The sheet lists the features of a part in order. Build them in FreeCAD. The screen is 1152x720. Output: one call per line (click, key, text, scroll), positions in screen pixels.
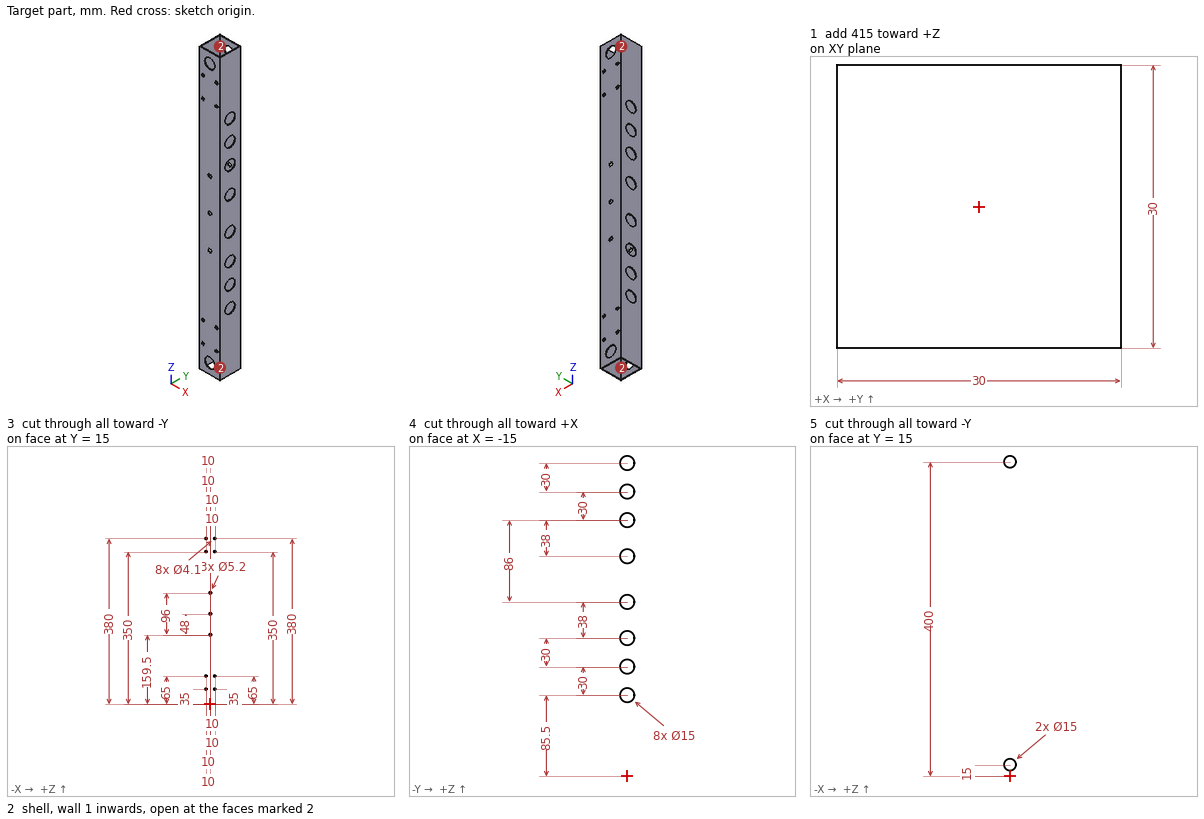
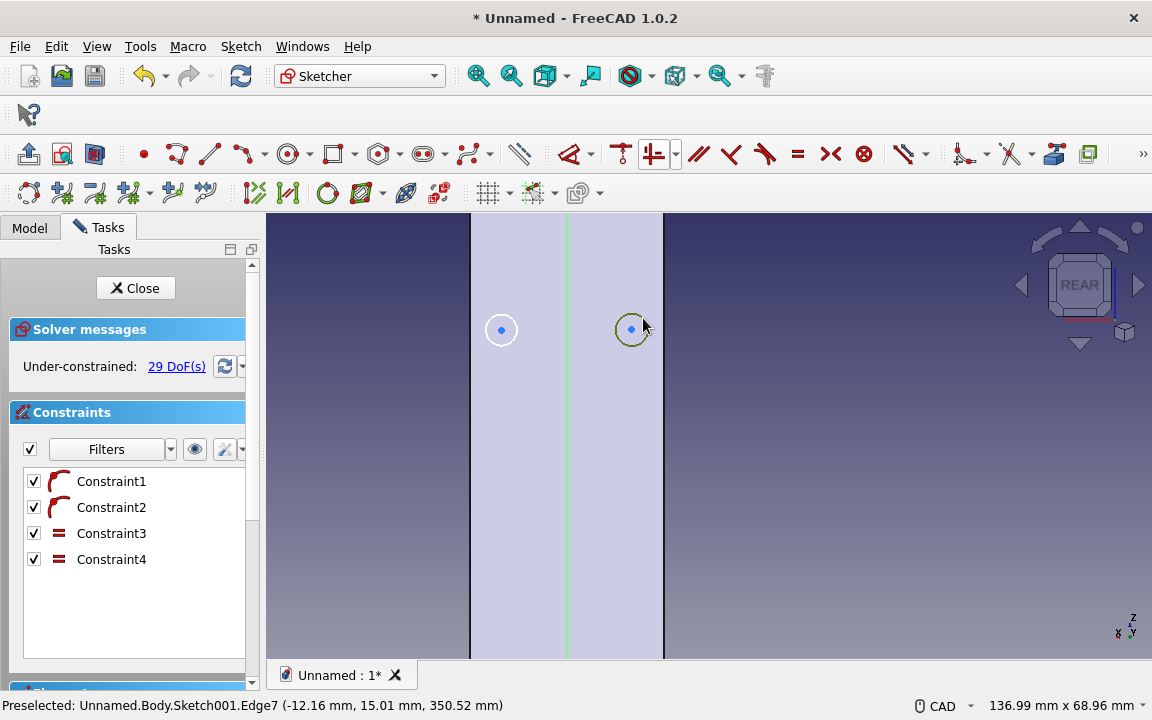
scroll(650, 322, down, 11)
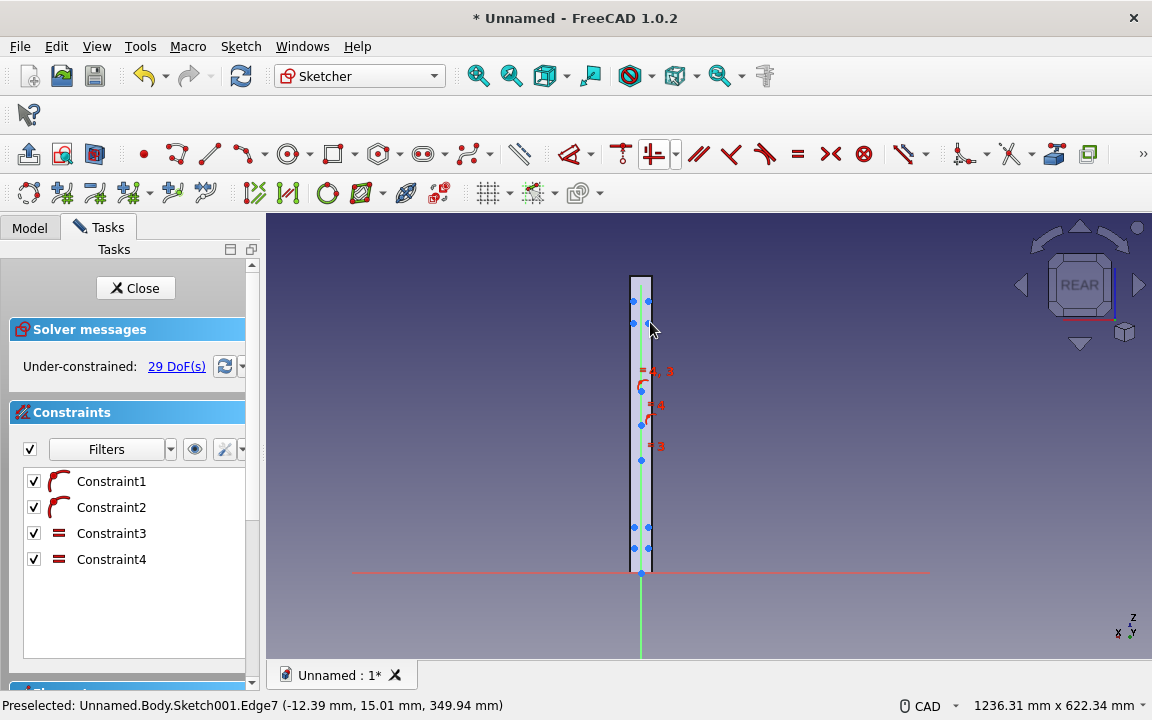
scroll(635, 526, up, 11)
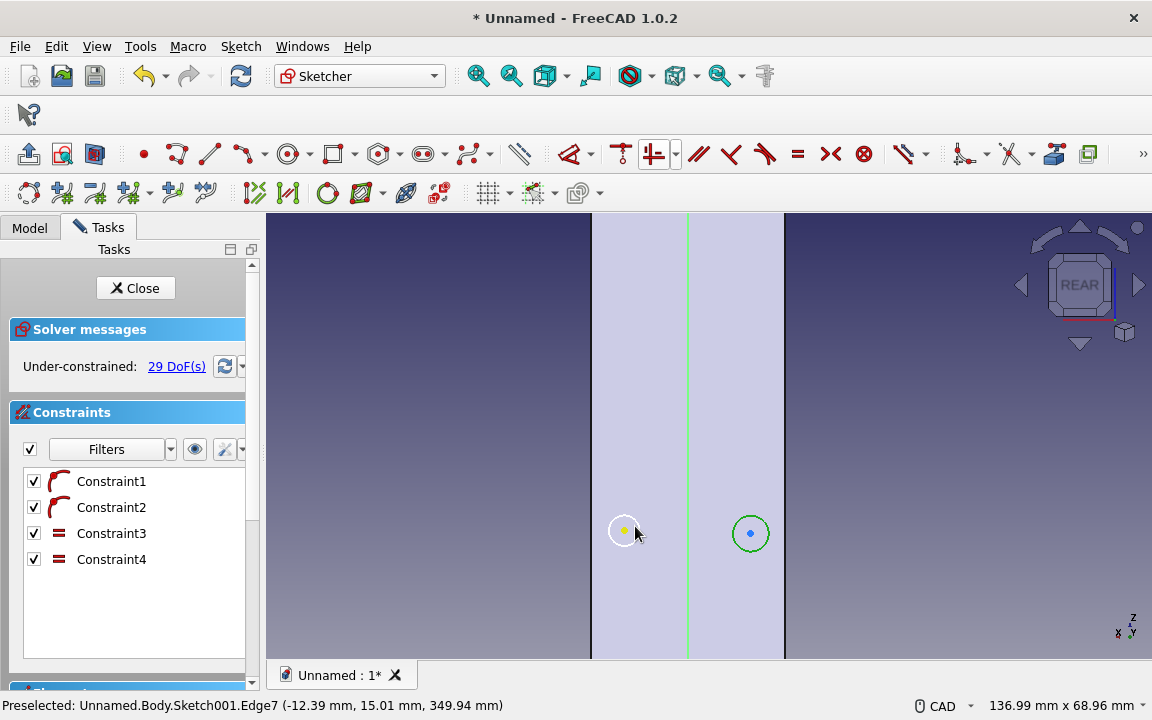
click(635, 520)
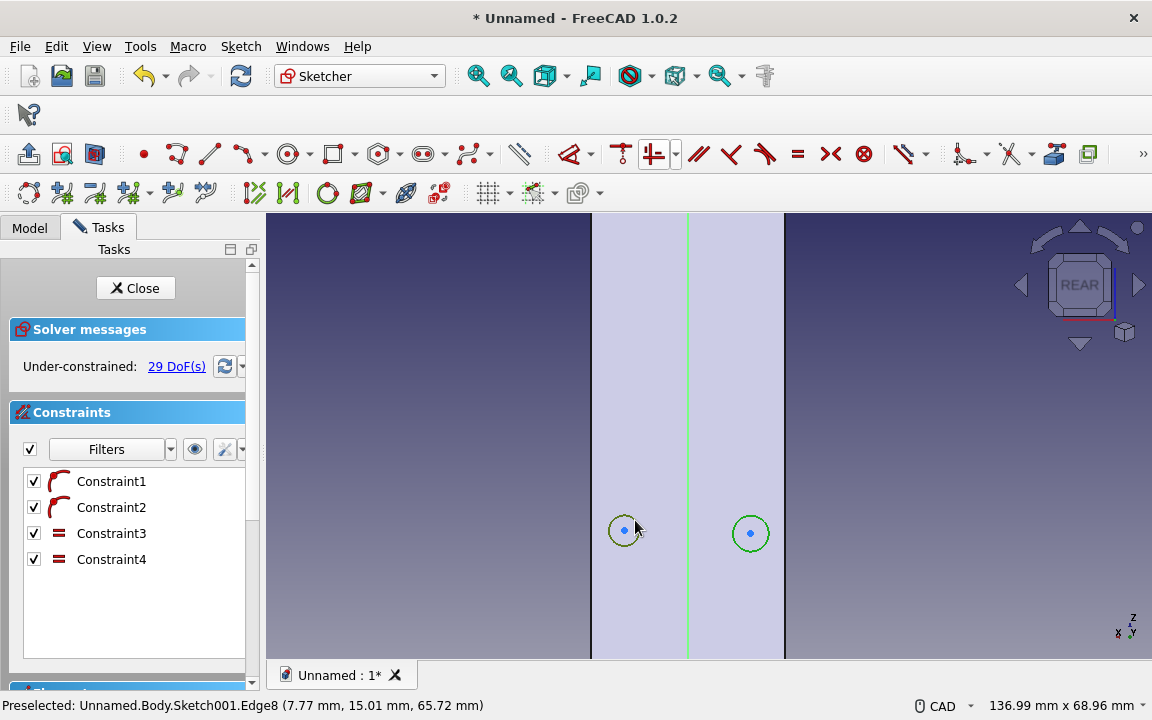
scroll(635, 526, down, 11)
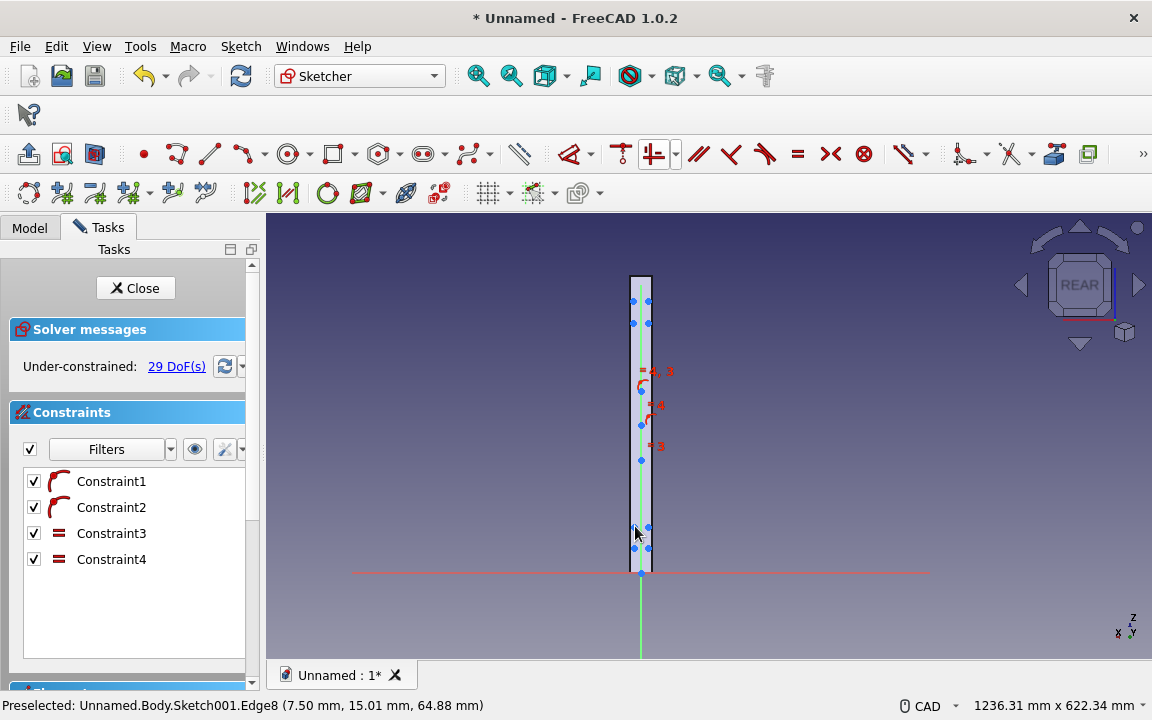
scroll(635, 322, up, 11)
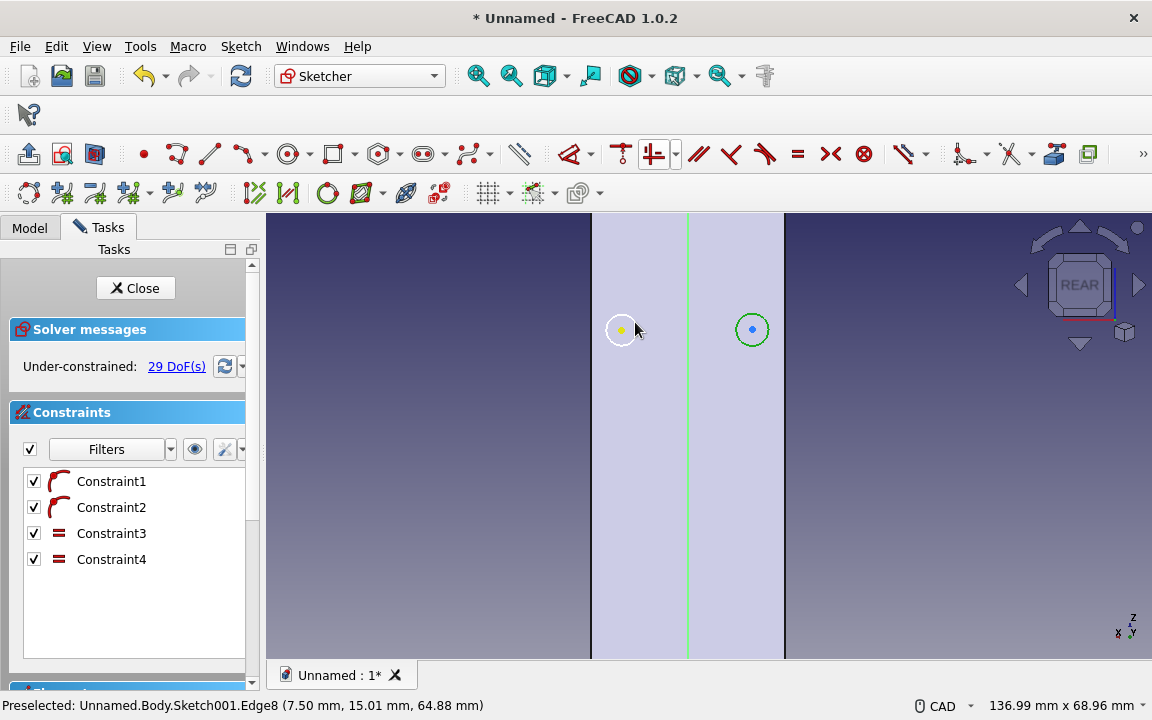
click(633, 319)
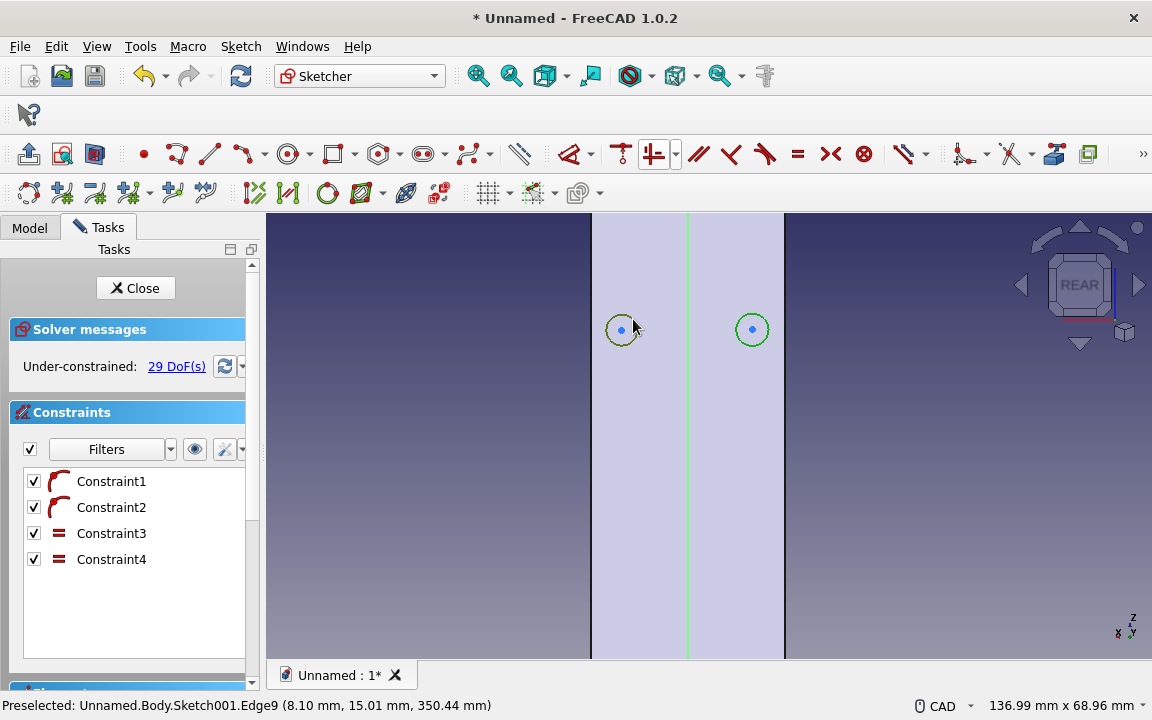
scroll(635, 322, down, 11)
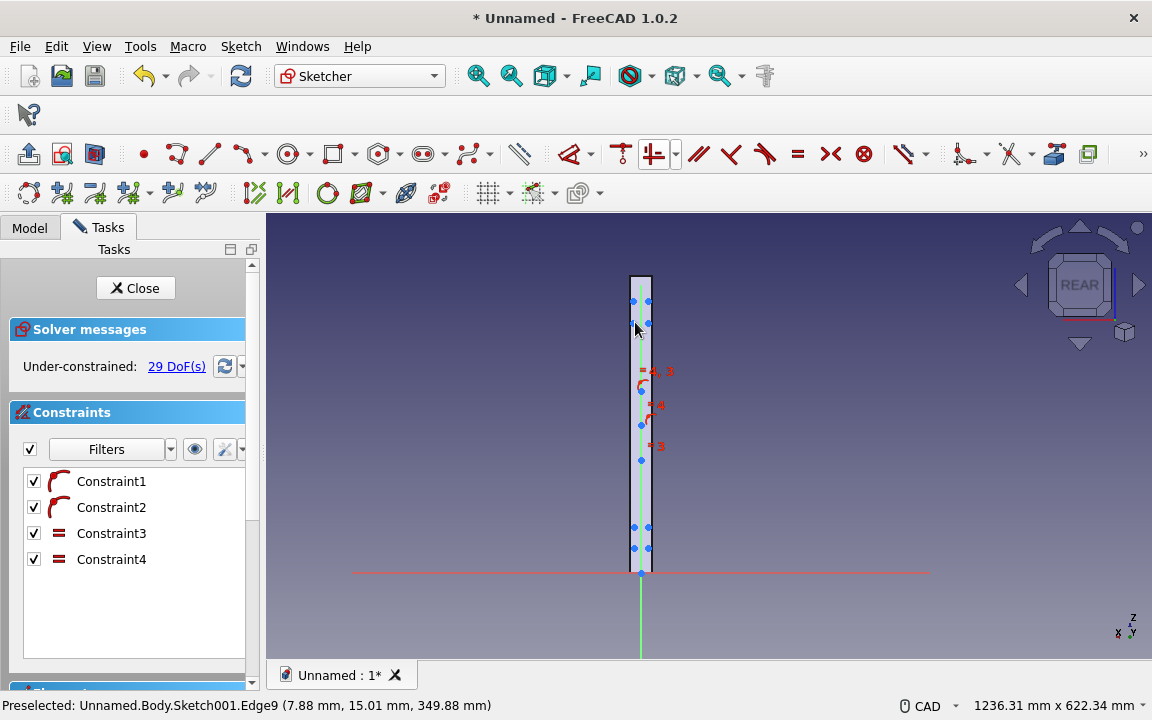
scroll(635, 547, up, 11)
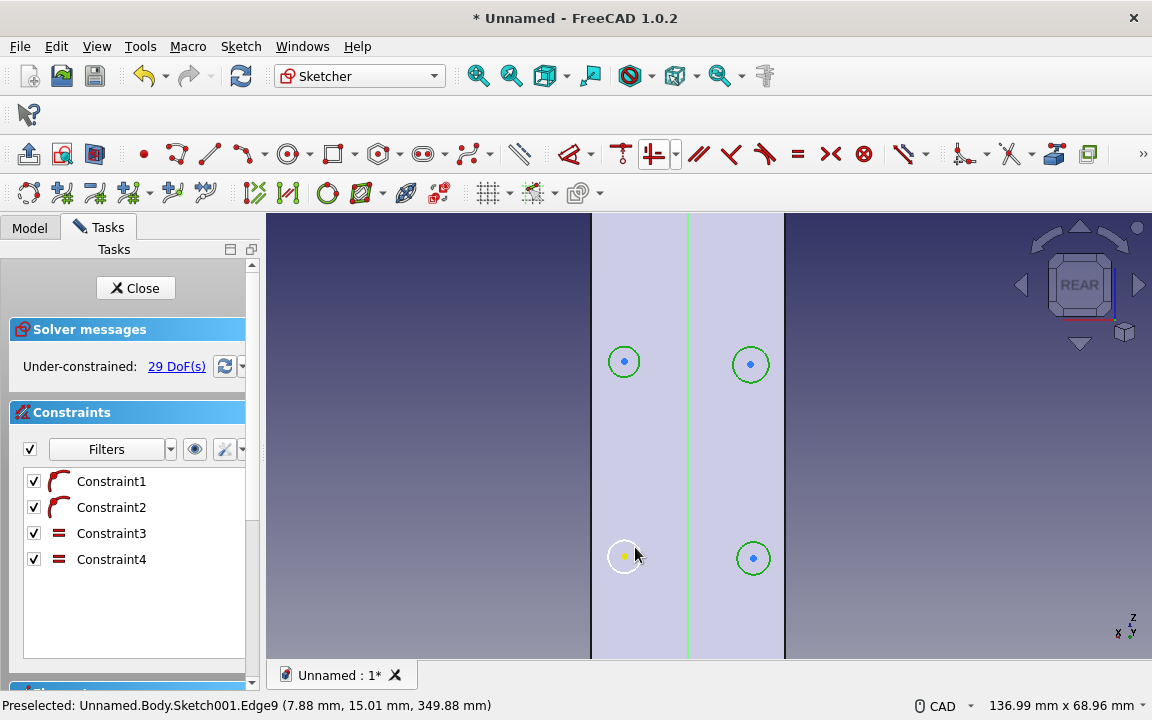
click(636, 545)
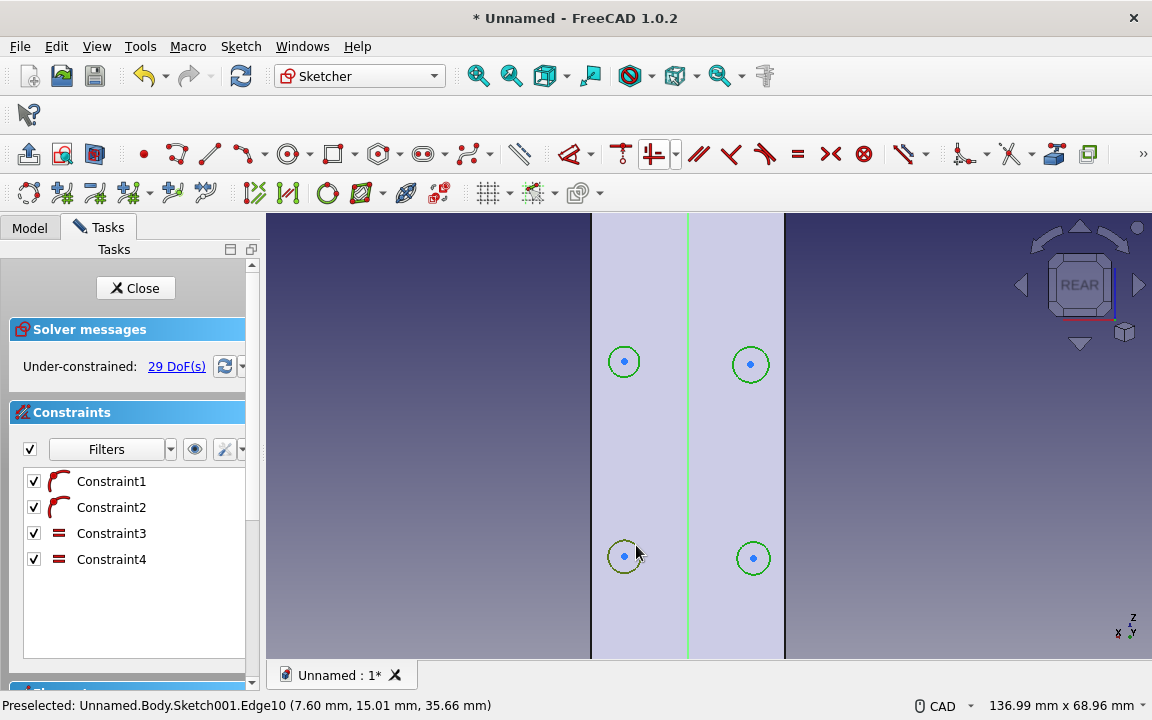
scroll(635, 547, down, 11)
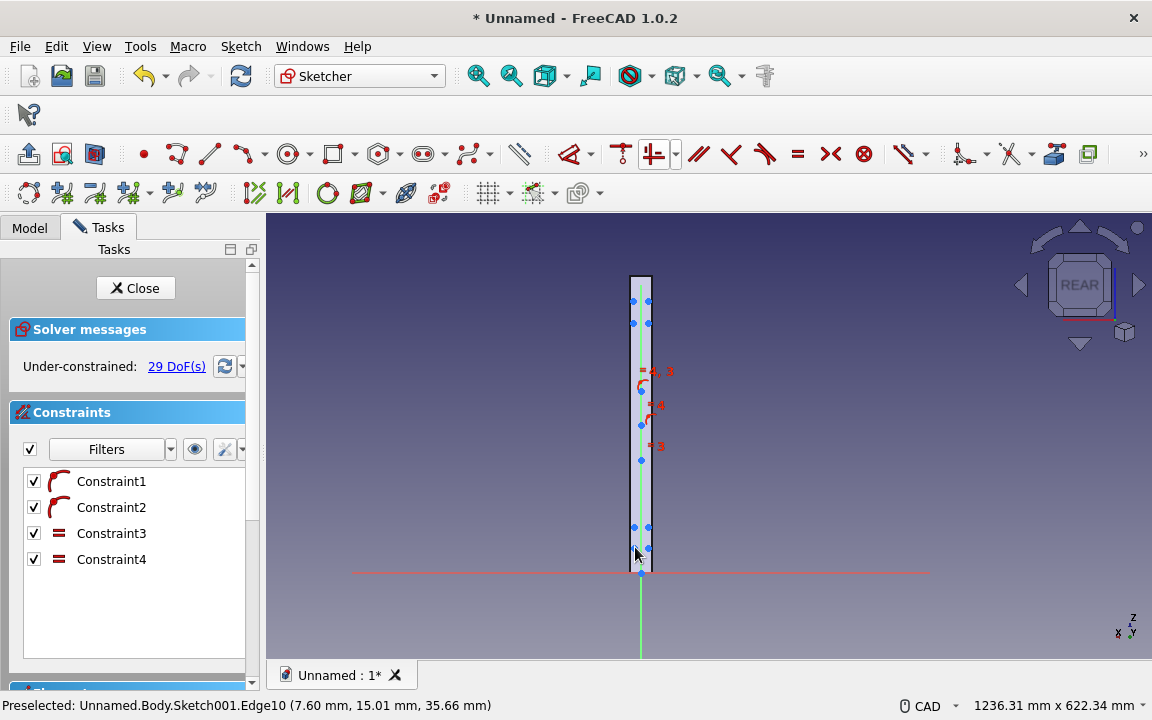
scroll(635, 300, up, 11)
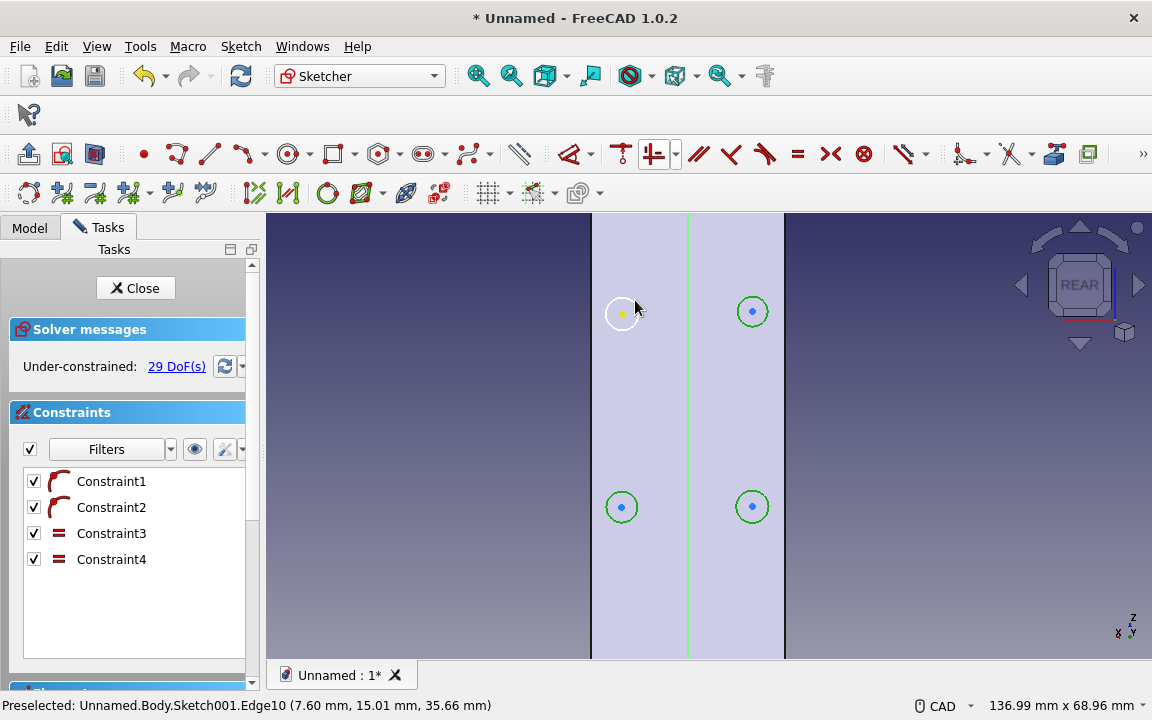
click(634, 302)